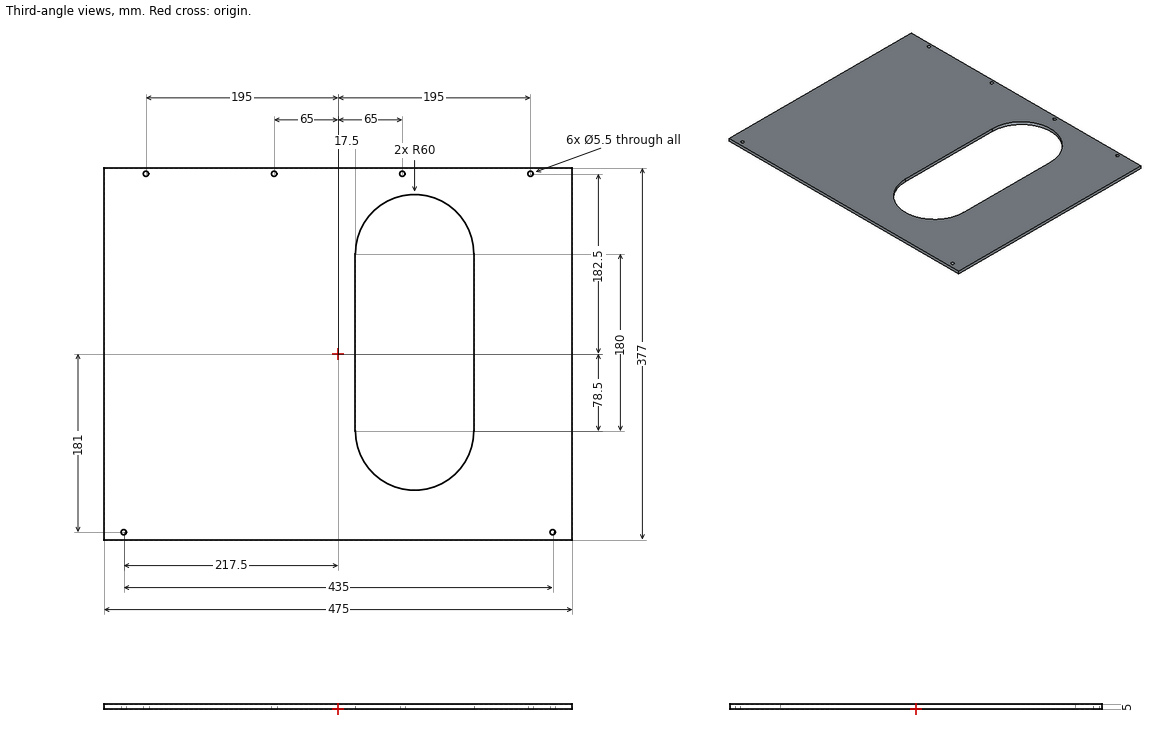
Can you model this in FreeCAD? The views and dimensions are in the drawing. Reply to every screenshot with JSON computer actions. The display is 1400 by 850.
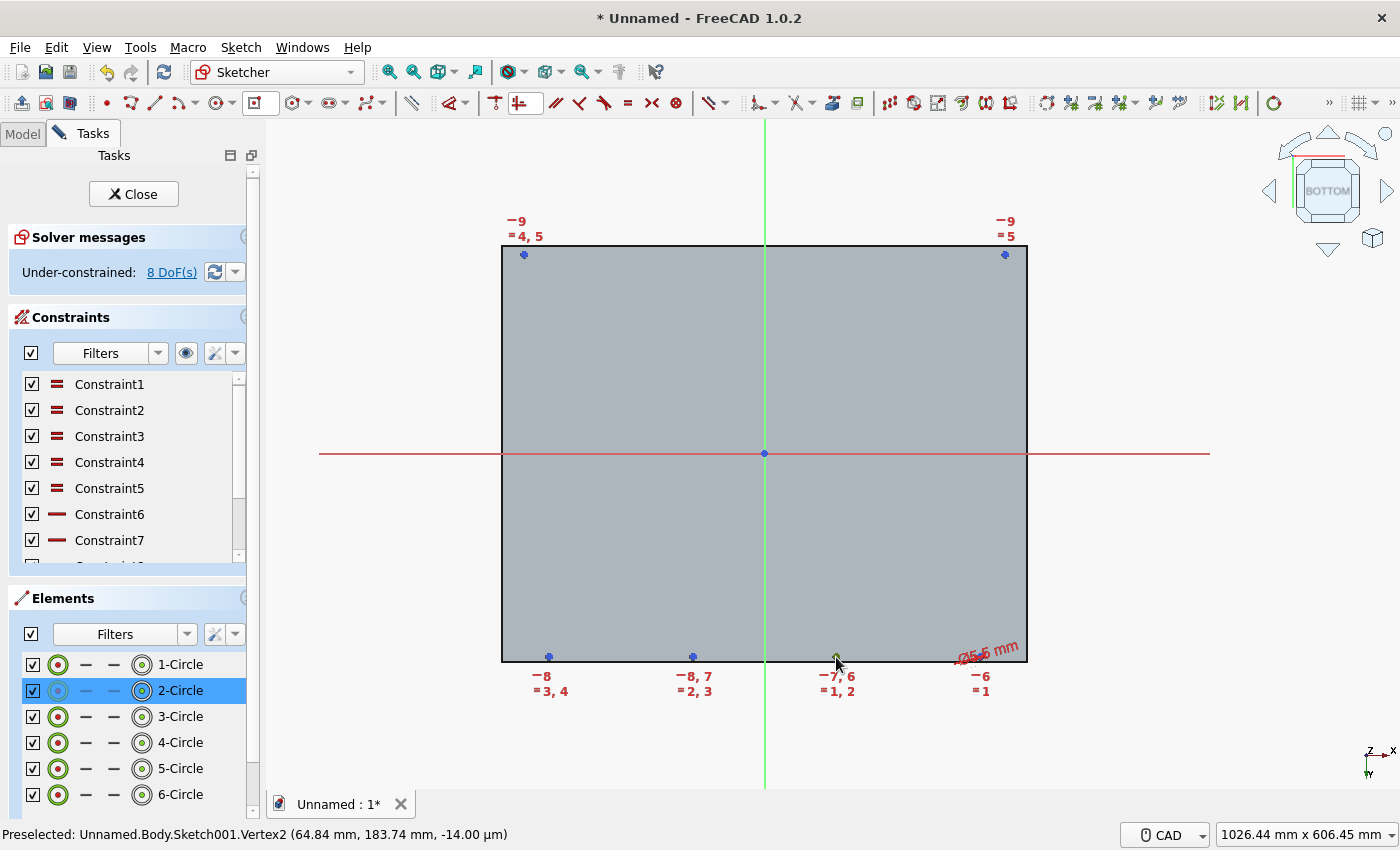
{"action": "key", "text": "l"}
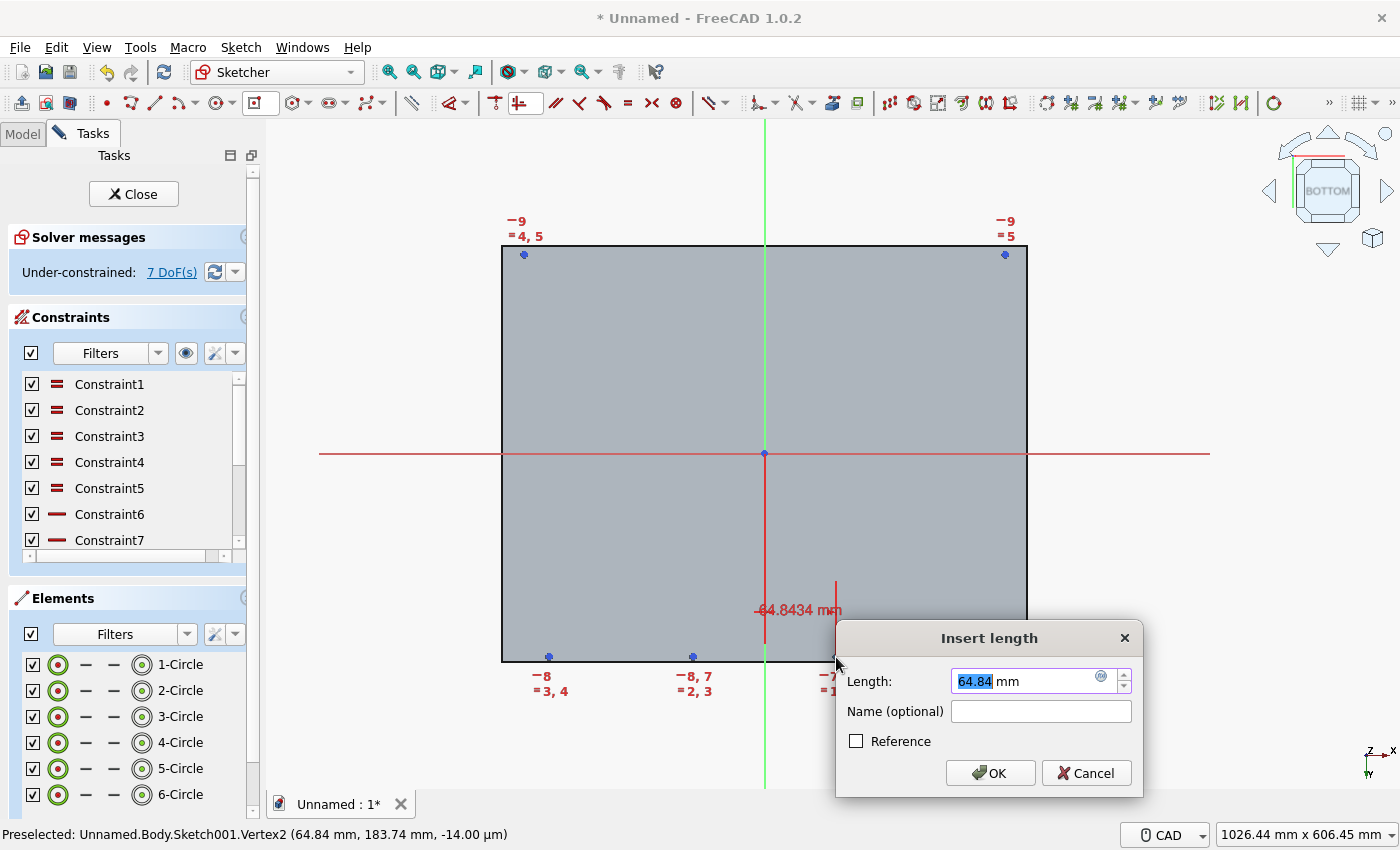
{"action": "type", "text": "65"}
{"action": "key", "text": "Return"}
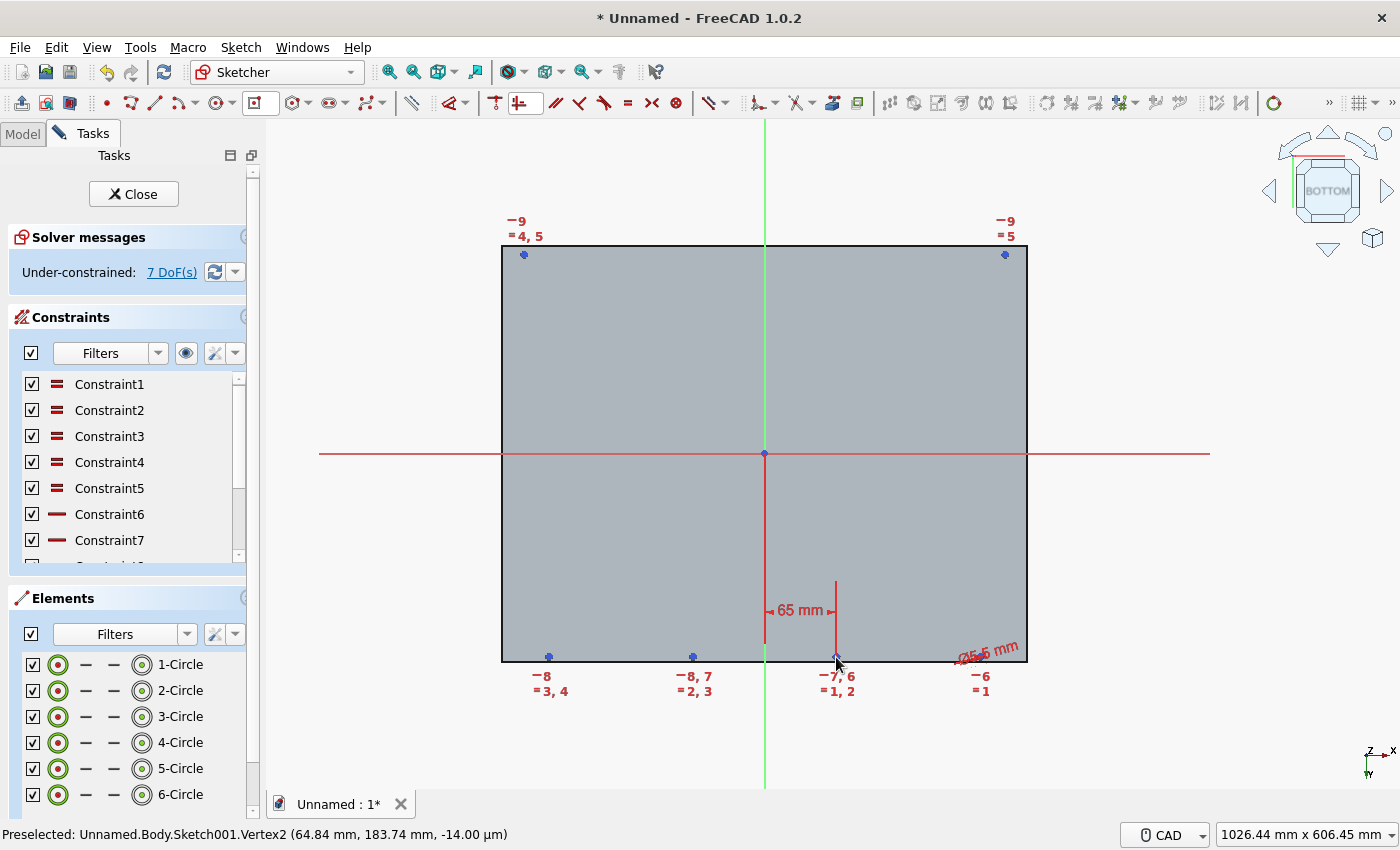
{"action": "left_click", "coordinate": [693, 657]}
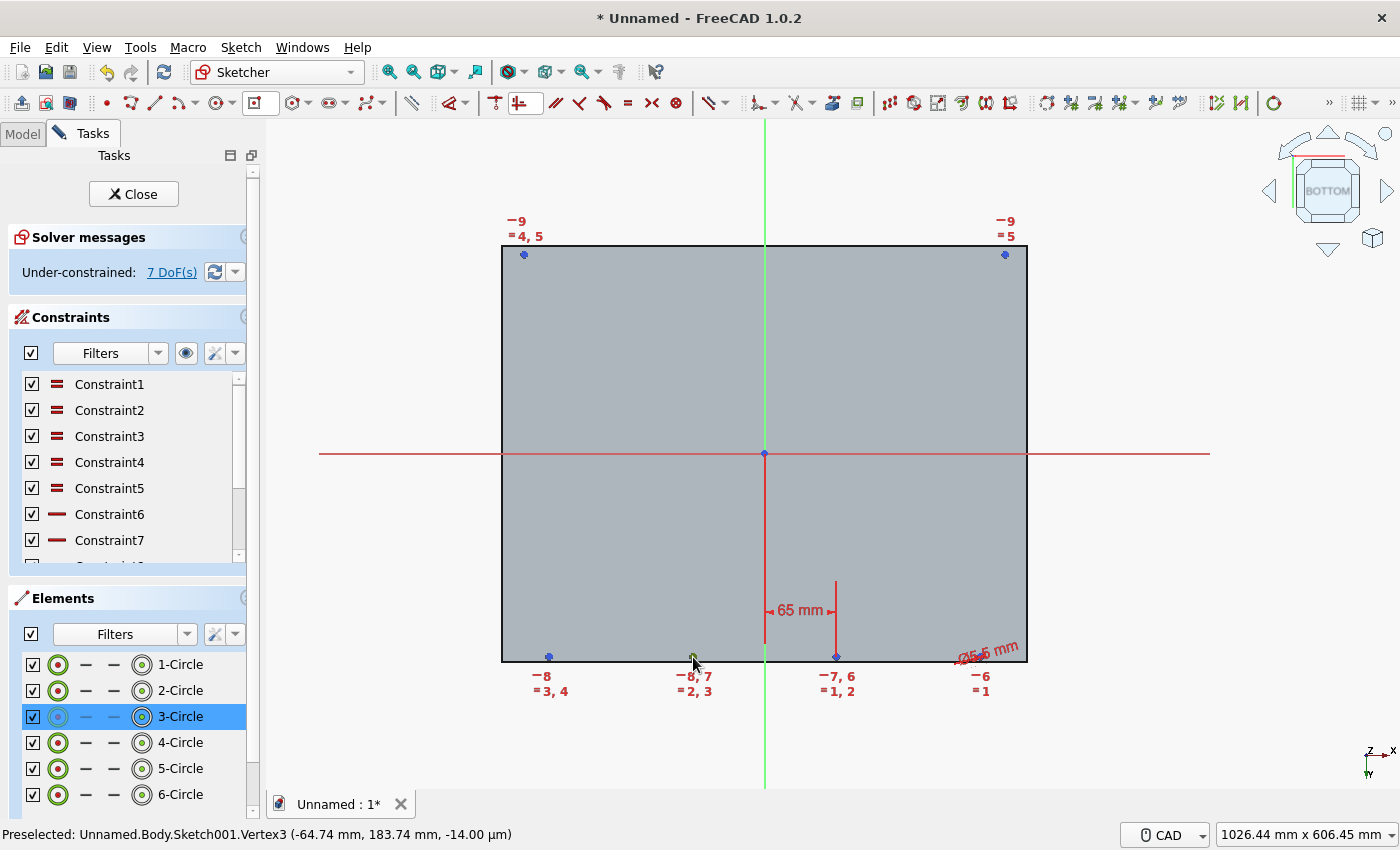
{"action": "key", "text": "l"}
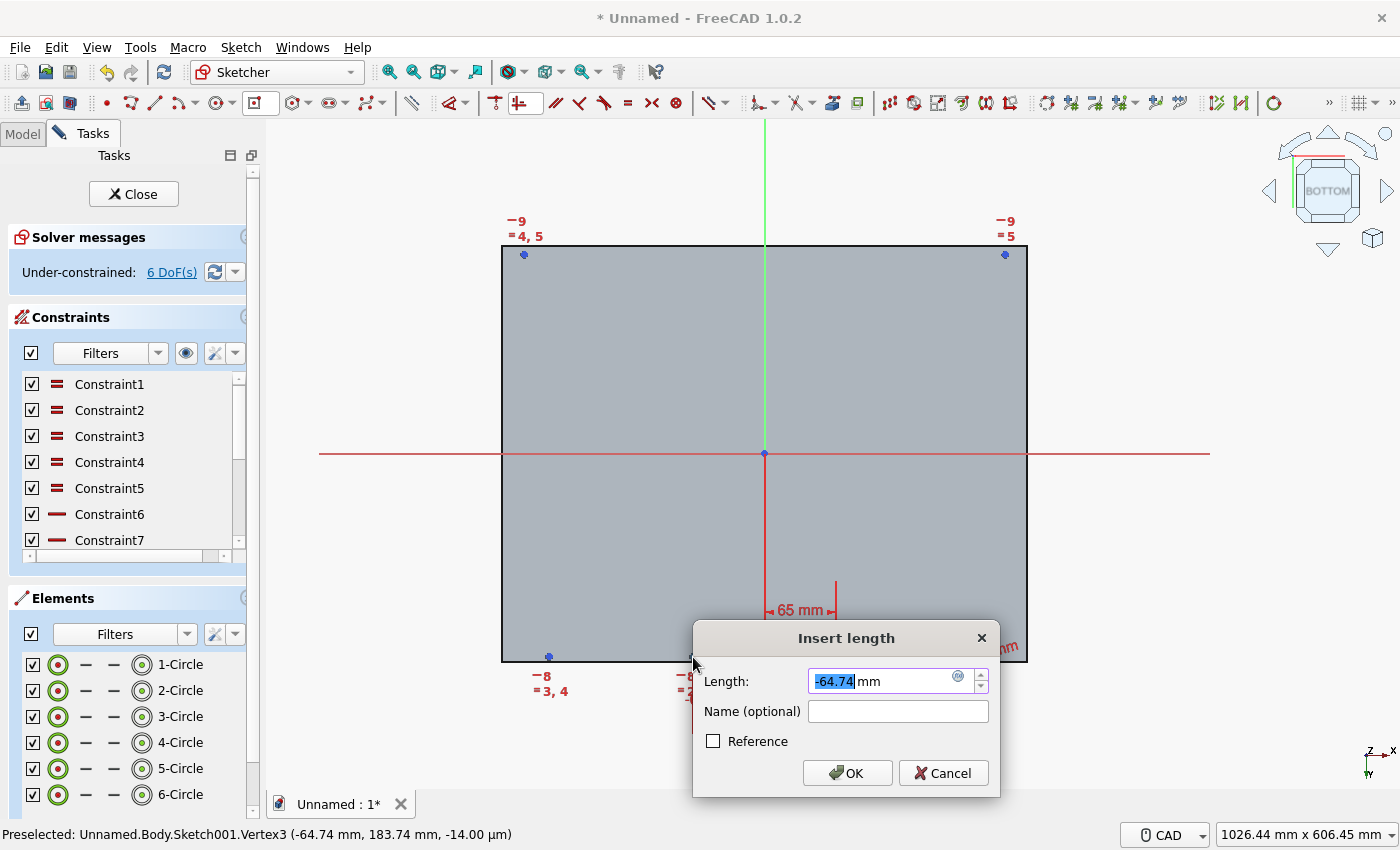
{"action": "type", "text": "-65"}
{"action": "key", "text": "Return"}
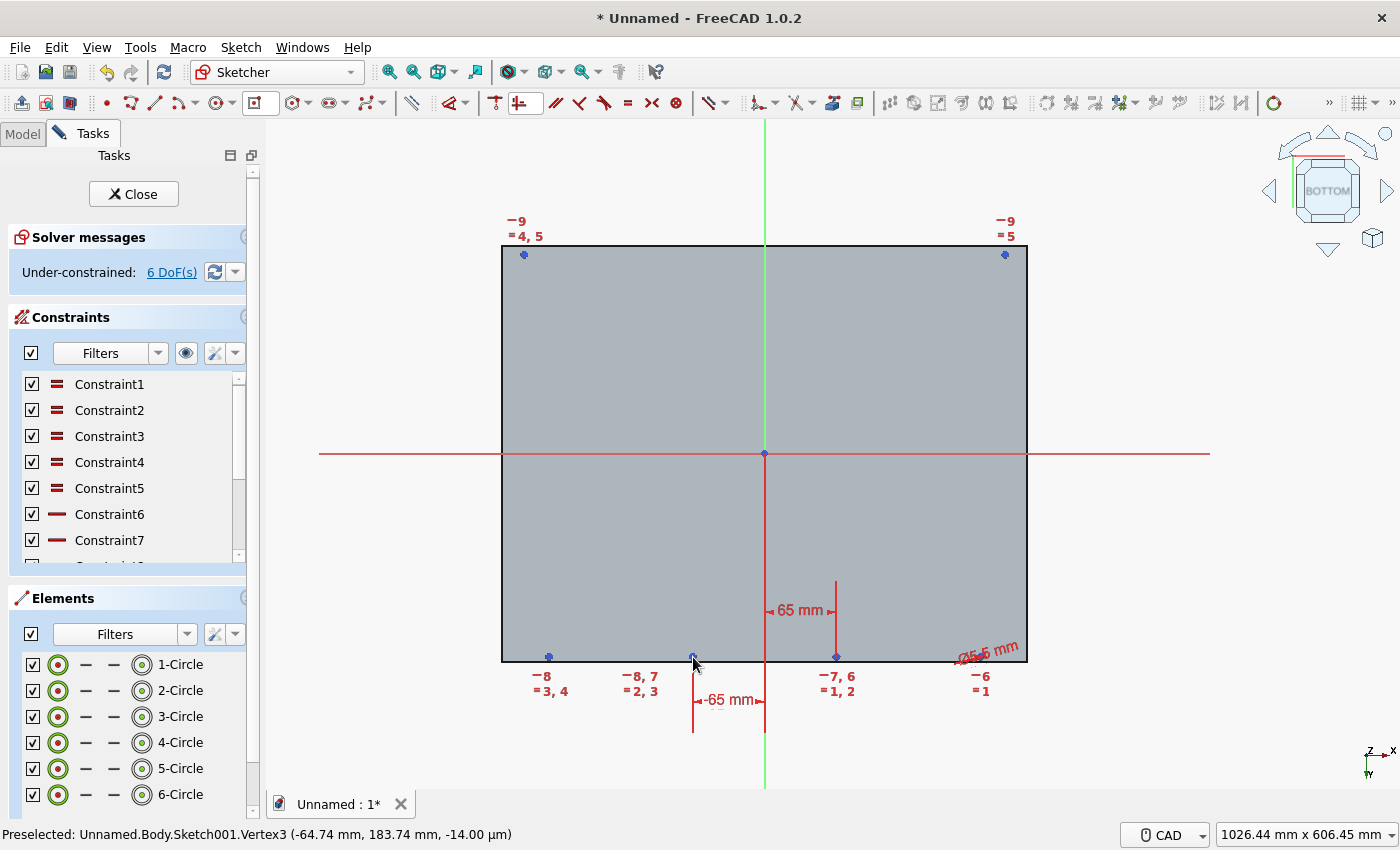
{"action": "left_click", "coordinate": [980, 657]}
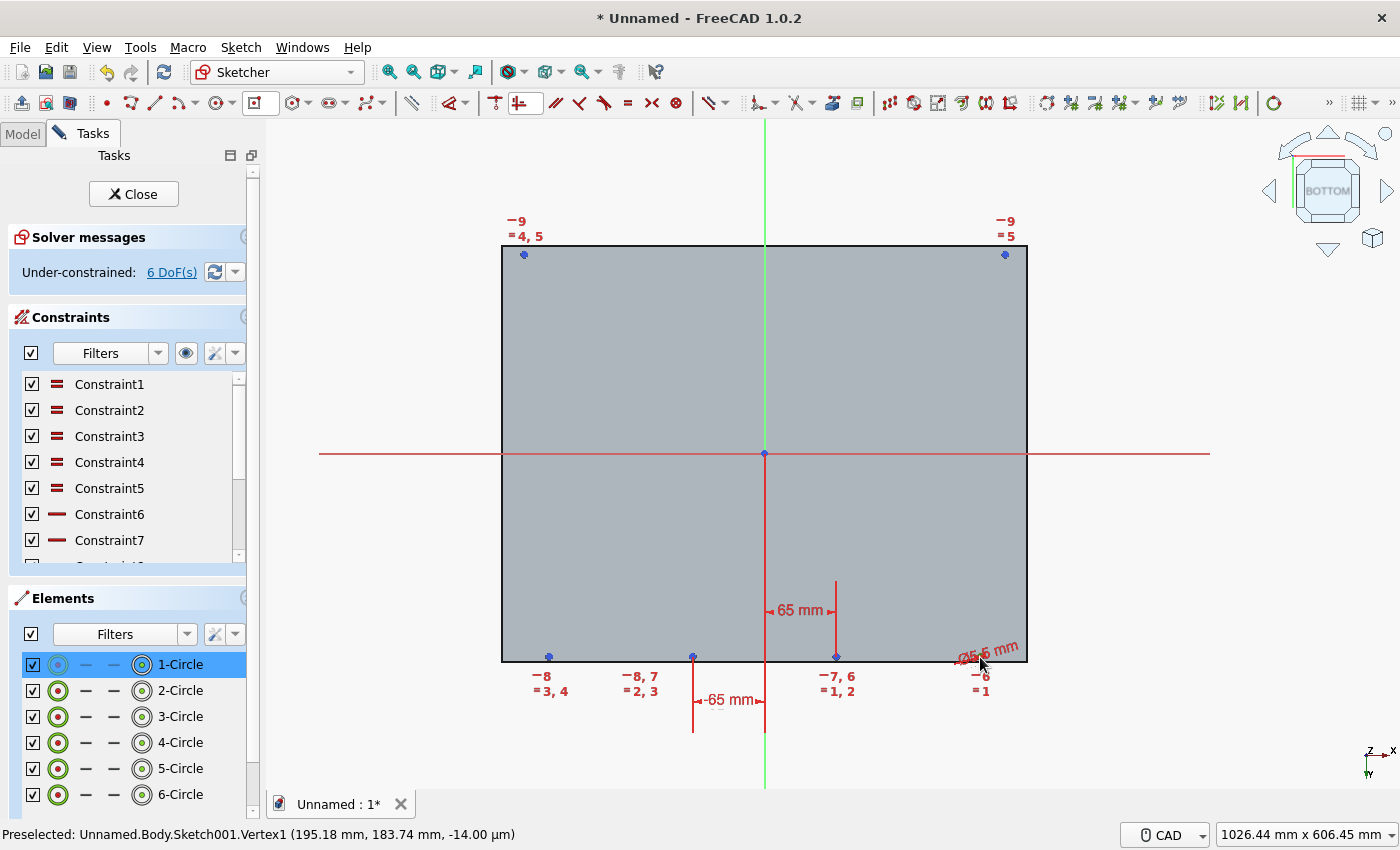
{"action": "key", "text": "l"}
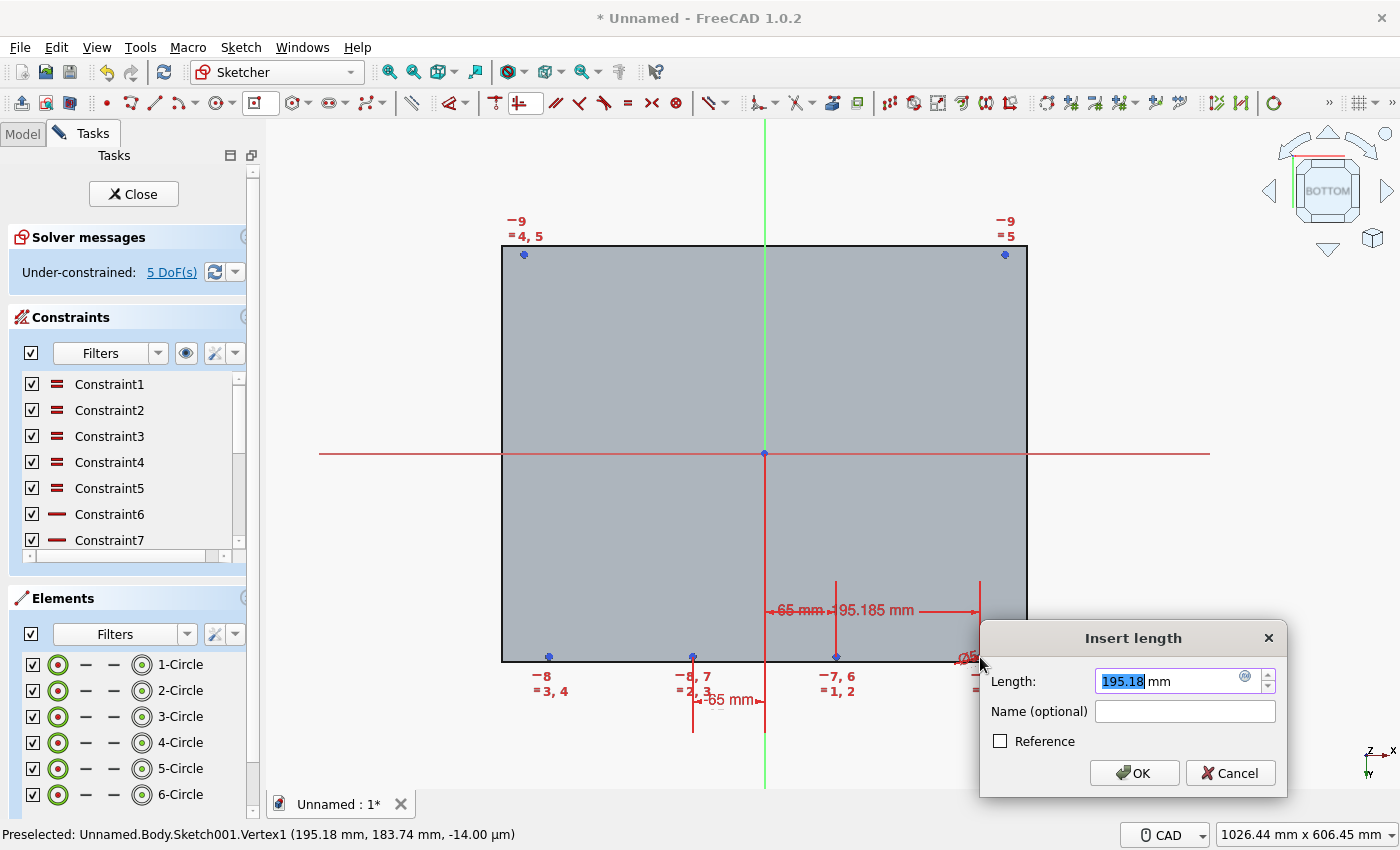
{"action": "type", "text": "195"}
{"action": "key", "text": "Return"}